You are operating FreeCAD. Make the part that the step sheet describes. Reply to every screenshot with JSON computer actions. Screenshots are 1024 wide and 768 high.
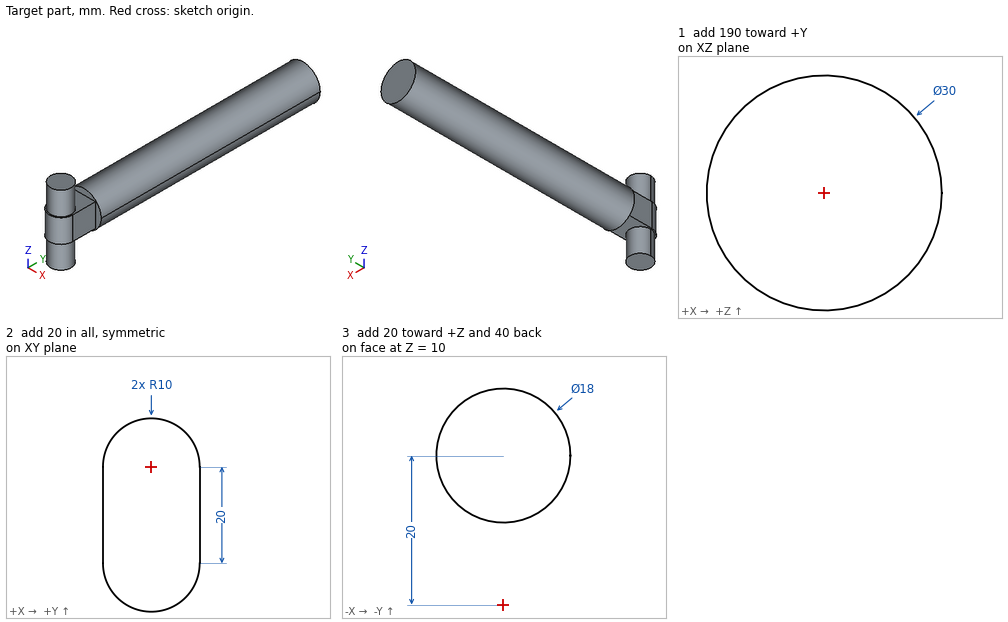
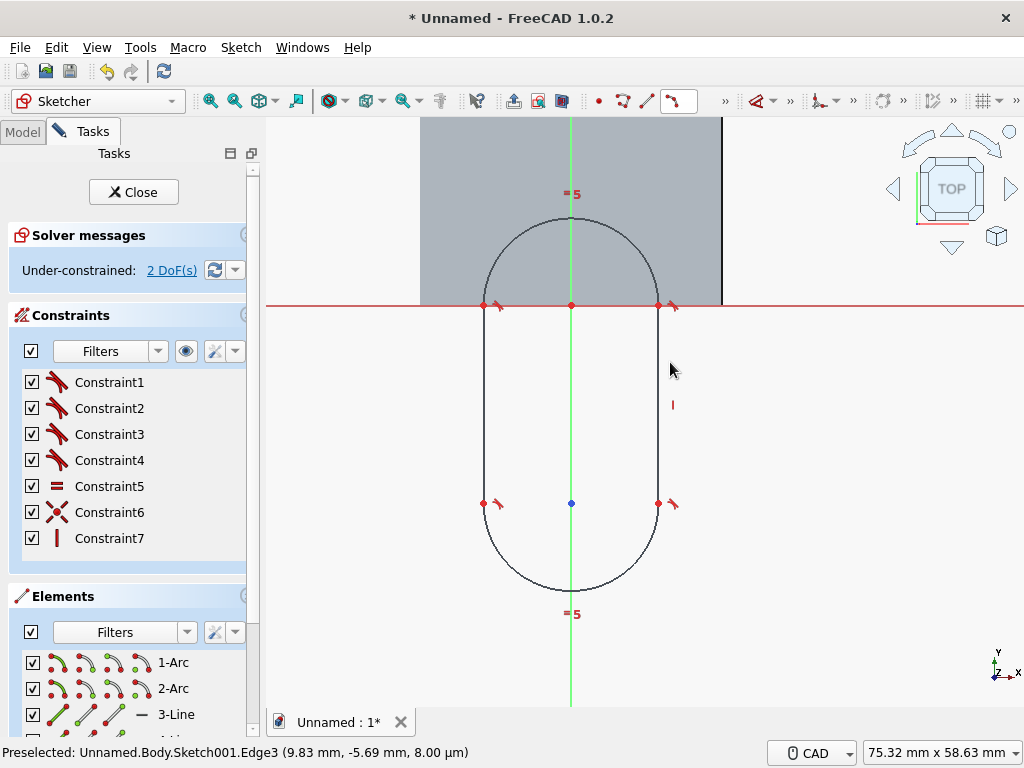
{"action": "key", "text": "d"}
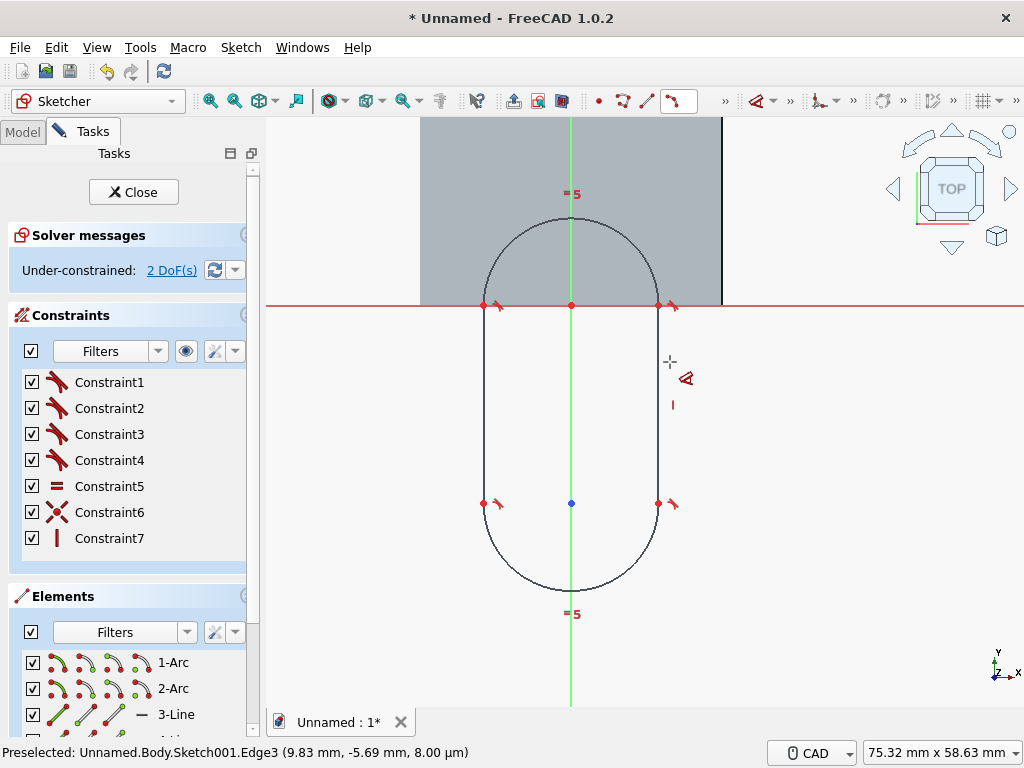
{"action": "left_click", "coordinate": [622, 235]}
{"action": "left_click", "coordinate": [641, 209]}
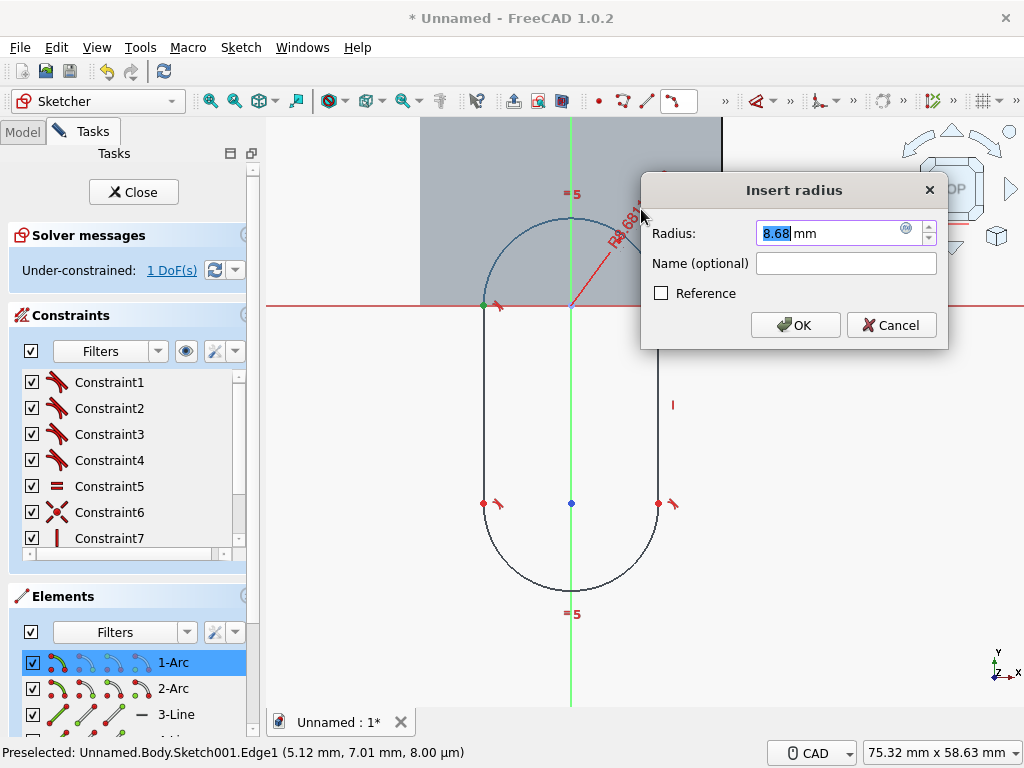
{"action": "type", "text": "10"}
{"action": "key", "text": "Return"}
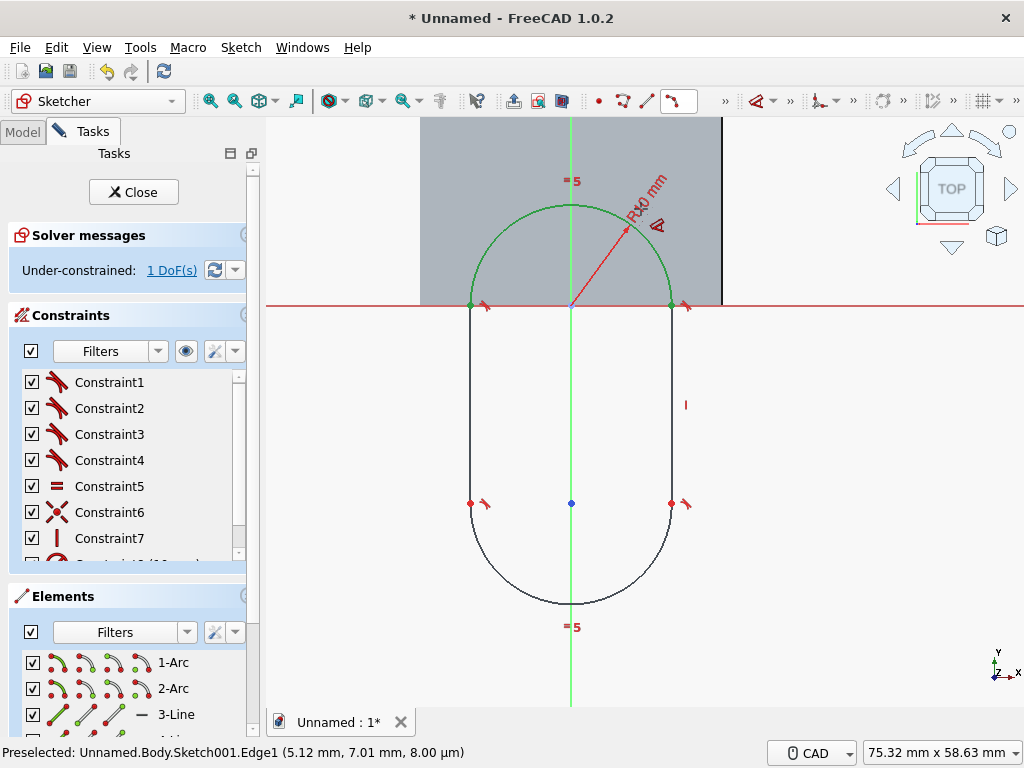
{"action": "left_click", "coordinate": [672, 365]}
{"action": "left_click", "coordinate": [706, 405]}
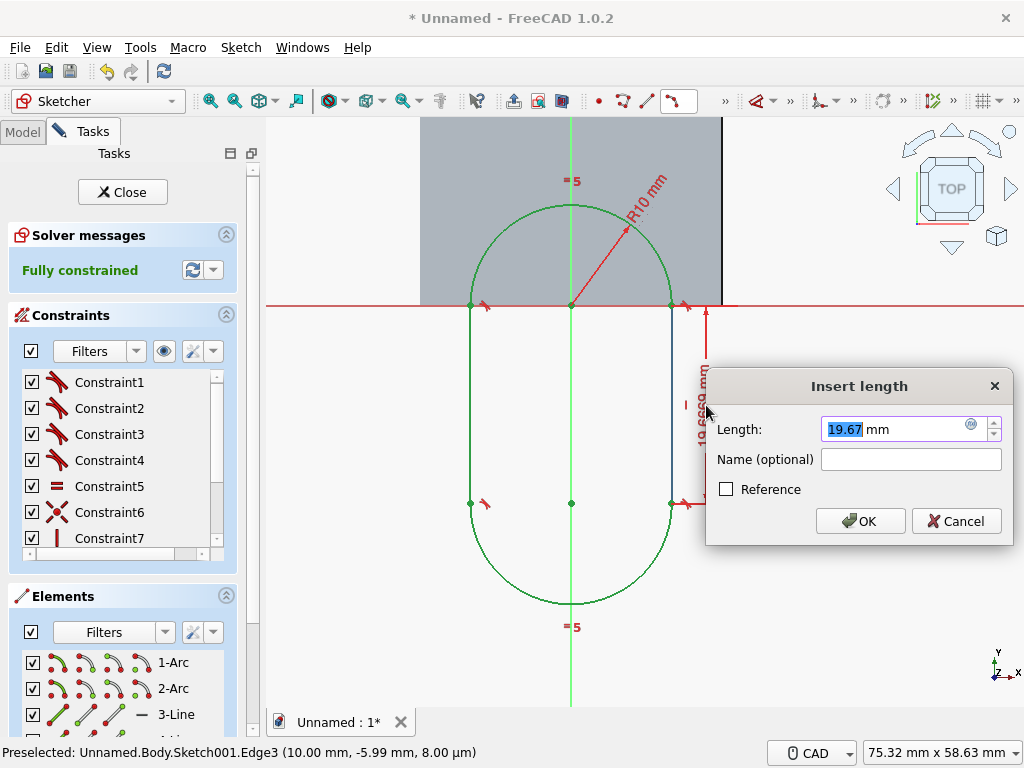
{"action": "type", "text": "20"}
{"action": "key", "text": "Return"}
{"action": "key", "text": "Escape"}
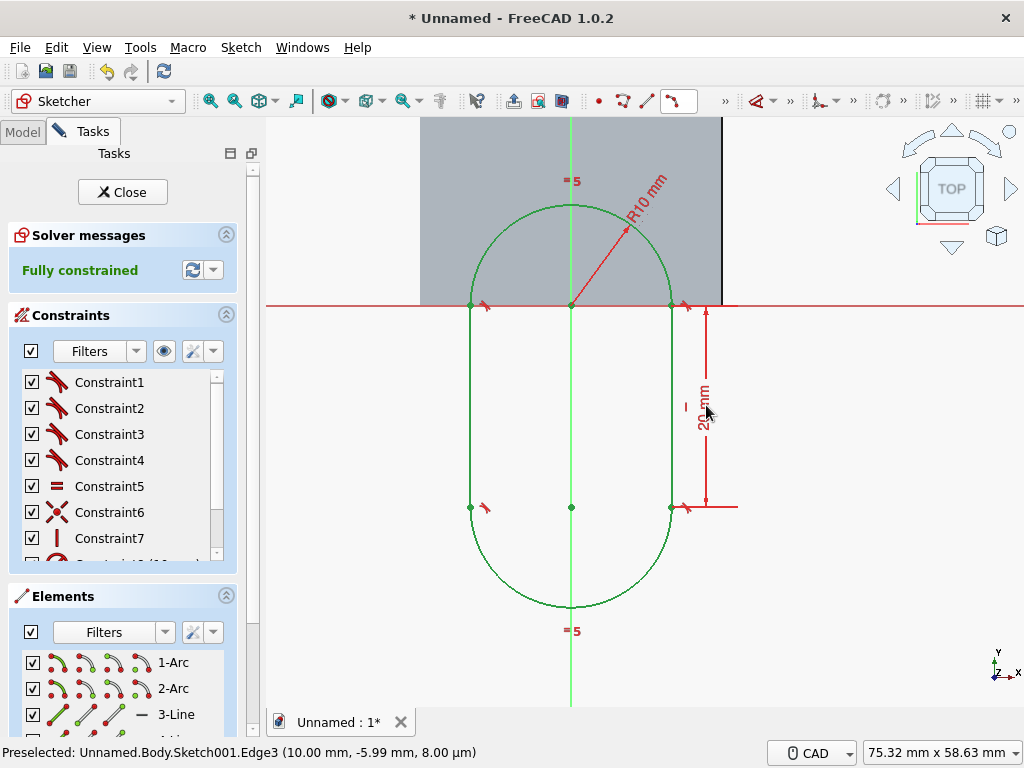
{"action": "left_click", "coordinate": [123, 192]}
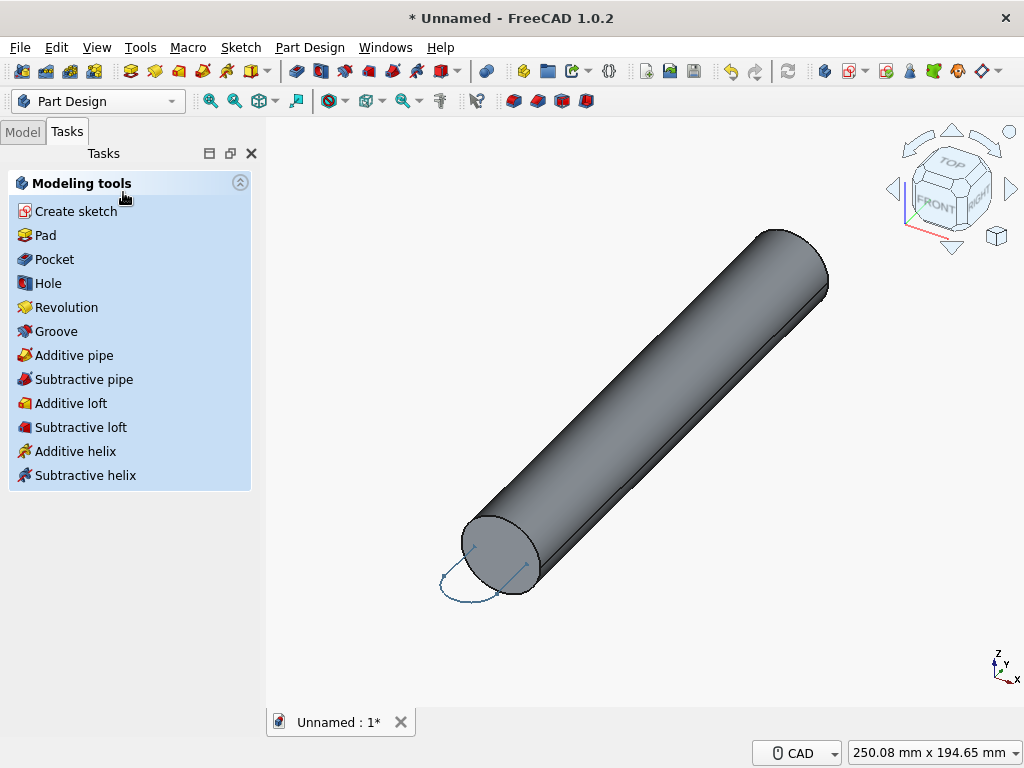
{"action": "left_click", "coordinate": [132, 72]}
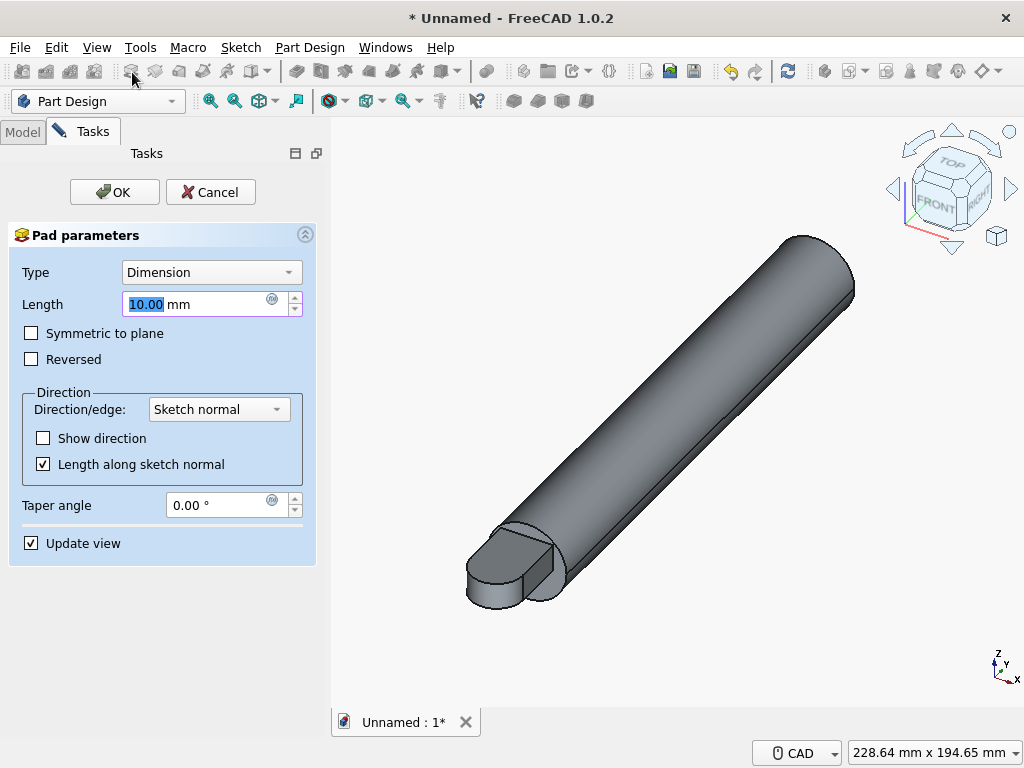
{"action": "type", "text": "20"}
{"action": "key", "text": "Tab"}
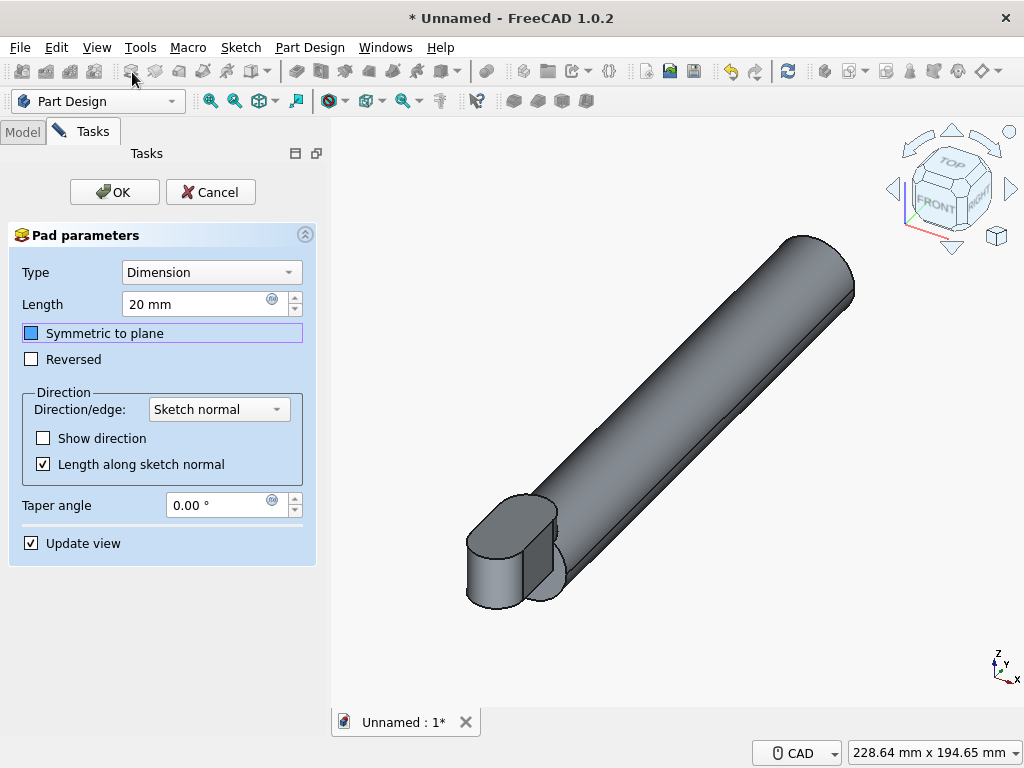
{"action": "left_click", "coordinate": [30, 333]}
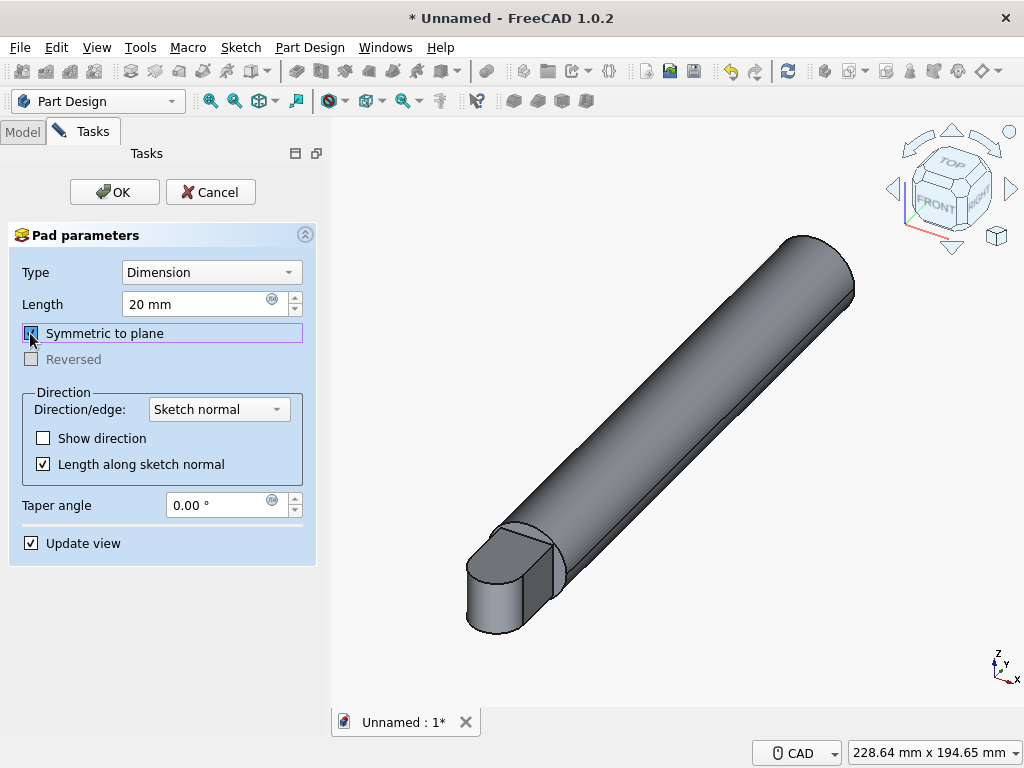
{"action": "left_click", "coordinate": [115, 192]}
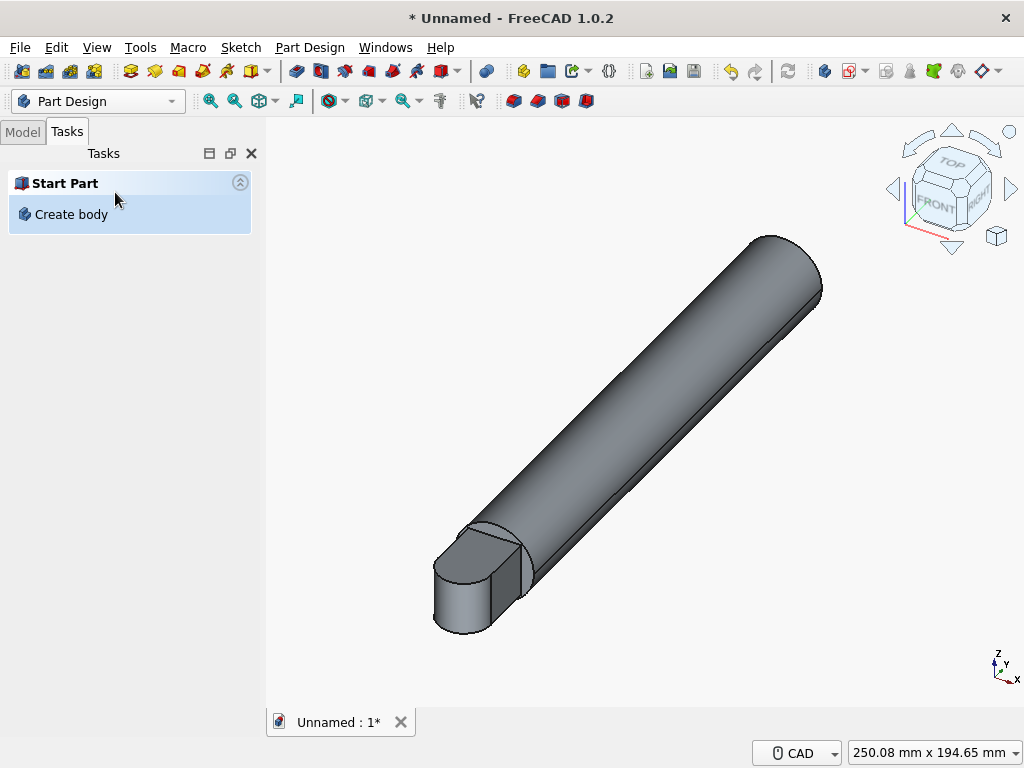
{"action": "left_click", "coordinate": [478, 552]}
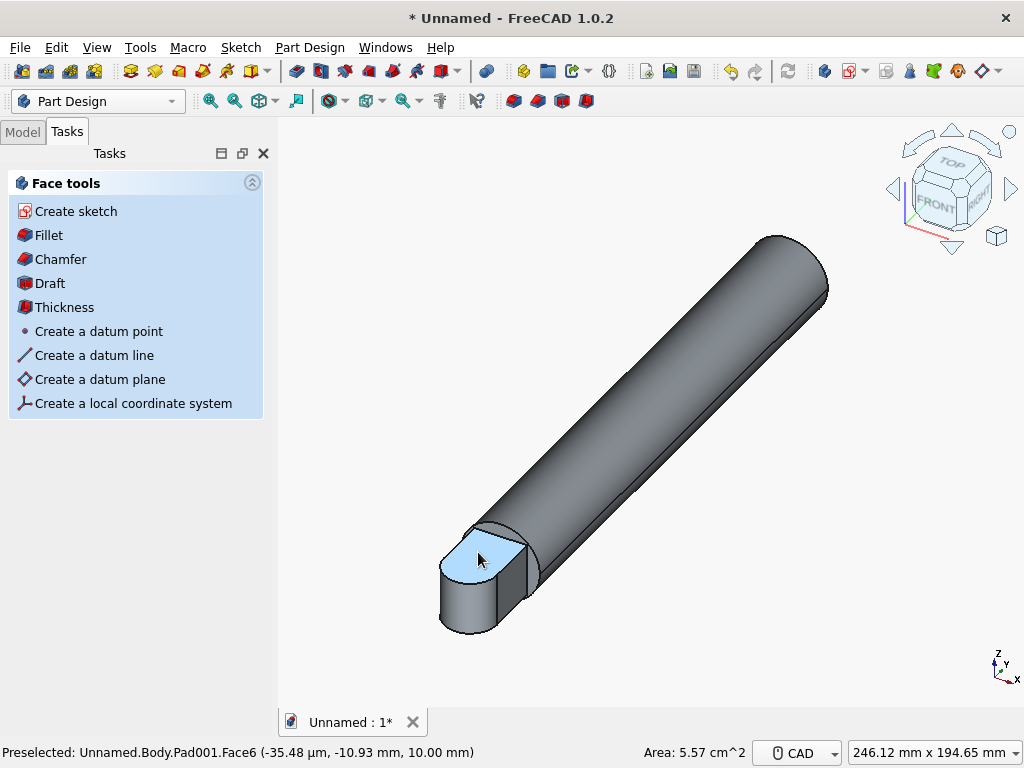
{"action": "left_click", "coordinate": [850, 72]}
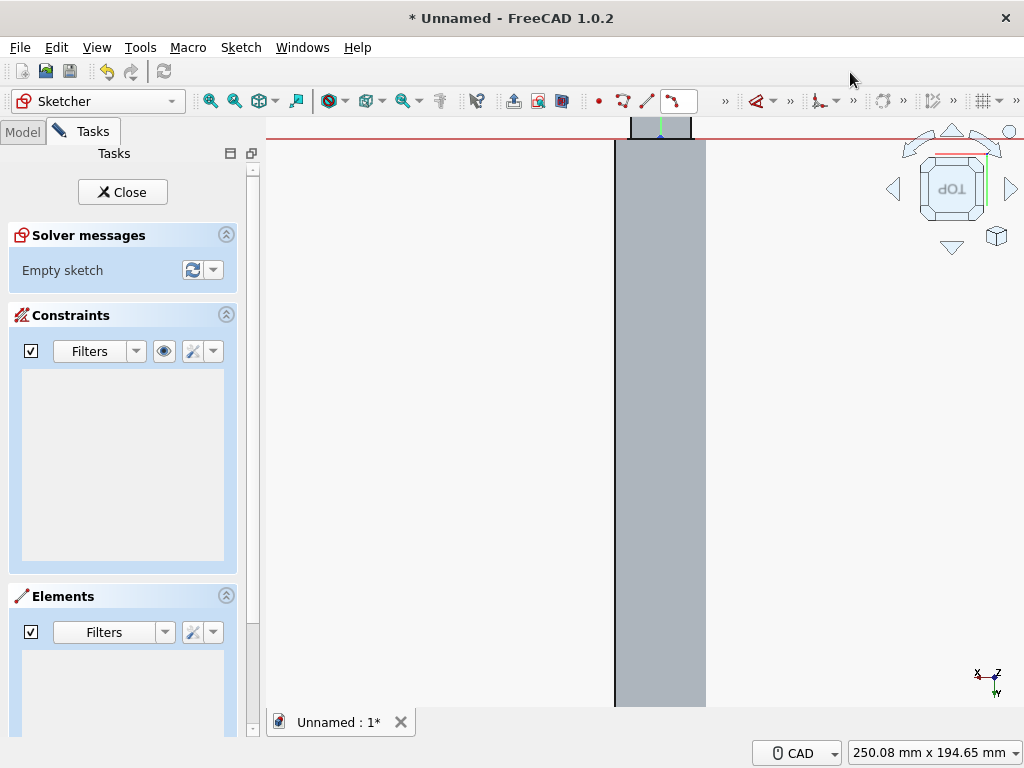
{"action": "key", "text": "q s"}